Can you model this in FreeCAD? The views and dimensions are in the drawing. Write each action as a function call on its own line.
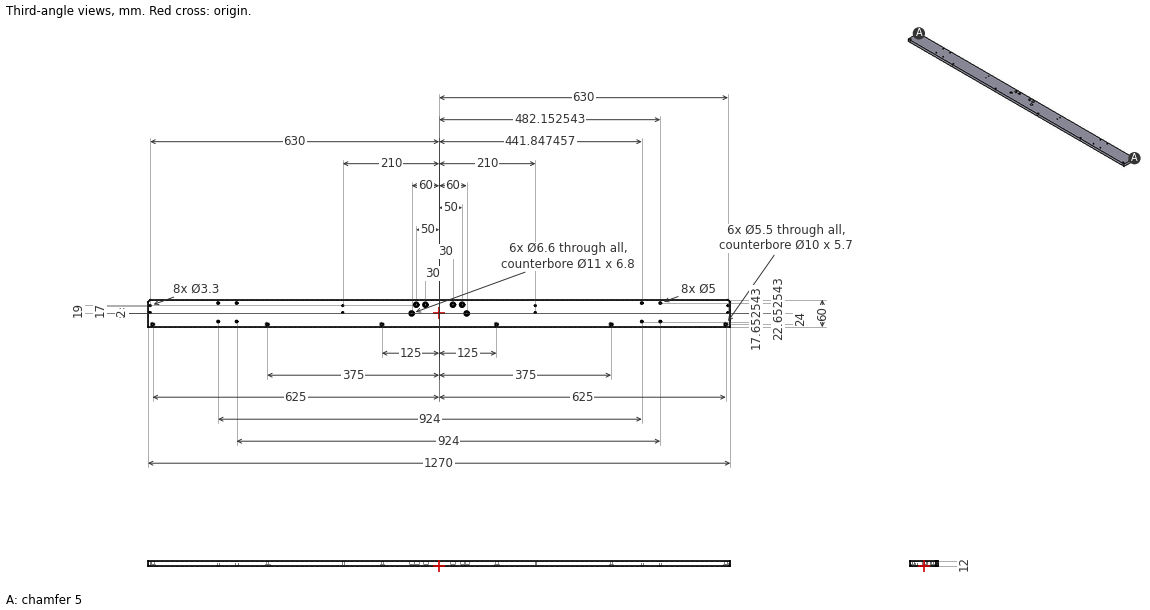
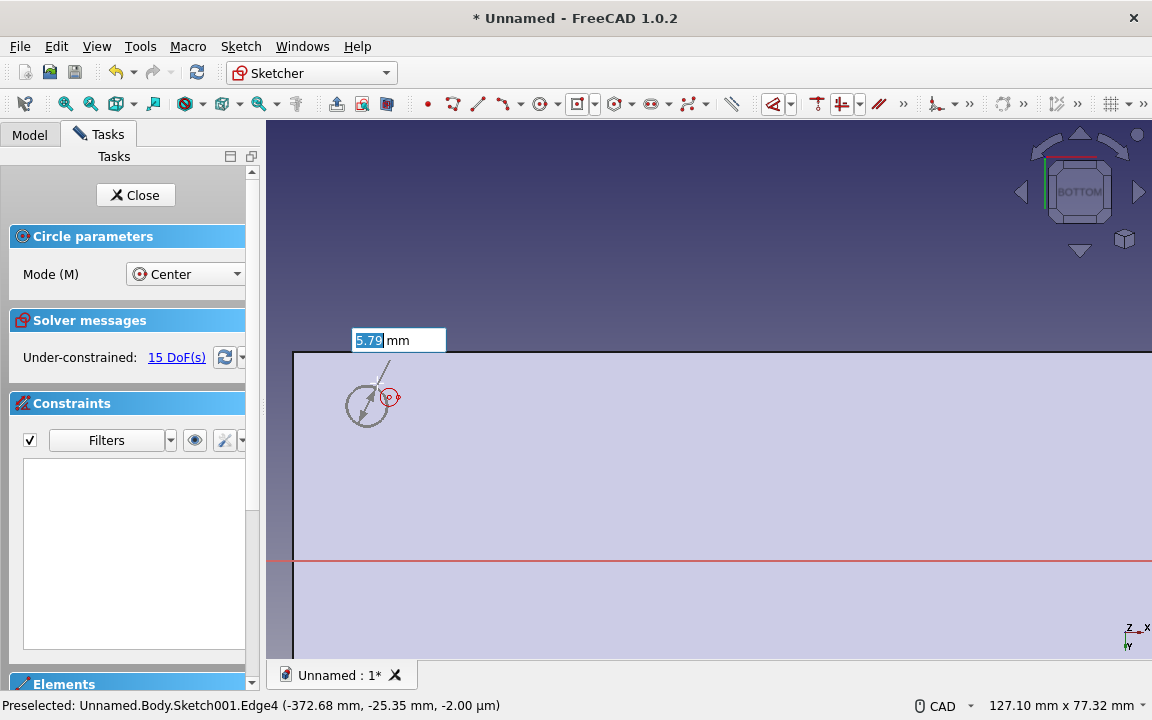
click(376, 380)
key(Escape)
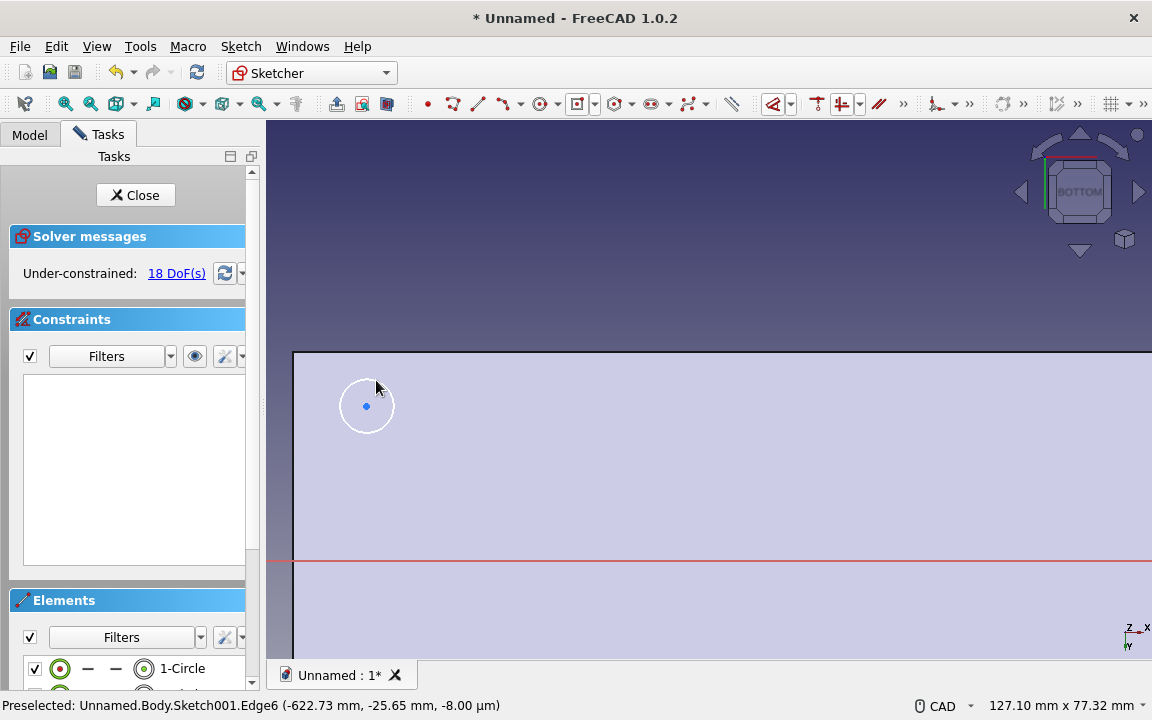
scroll(376, 384, down, 14)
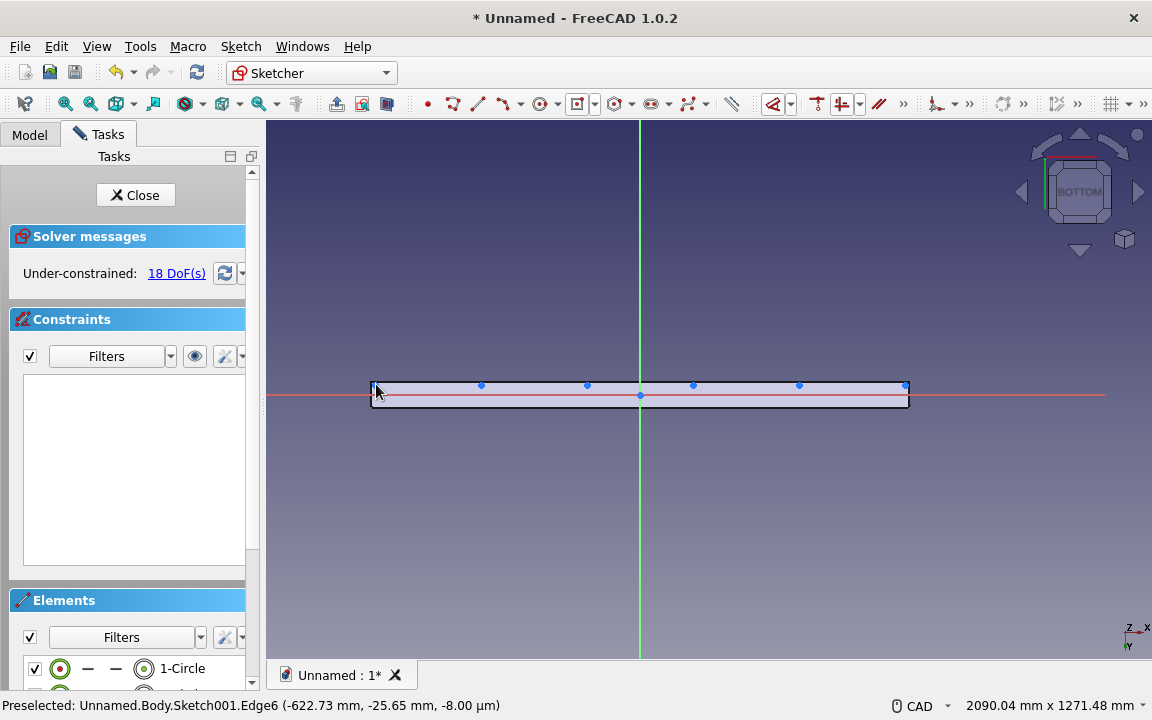
scroll(906, 384, up, 12)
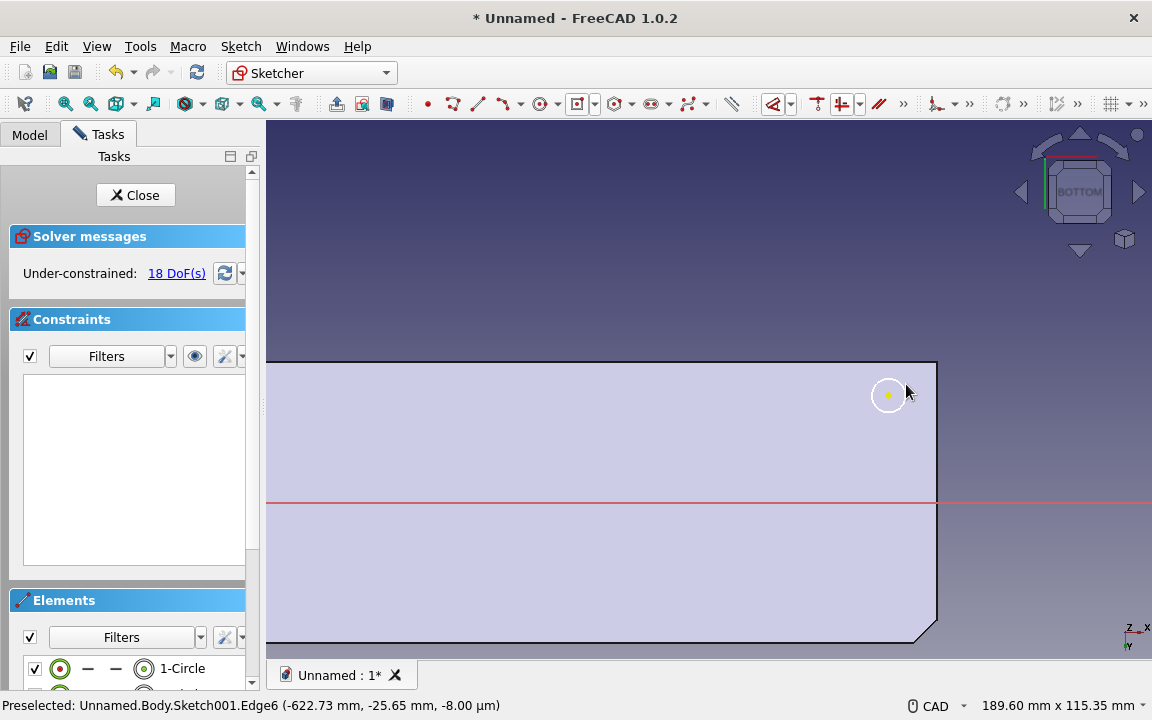
click(901, 384)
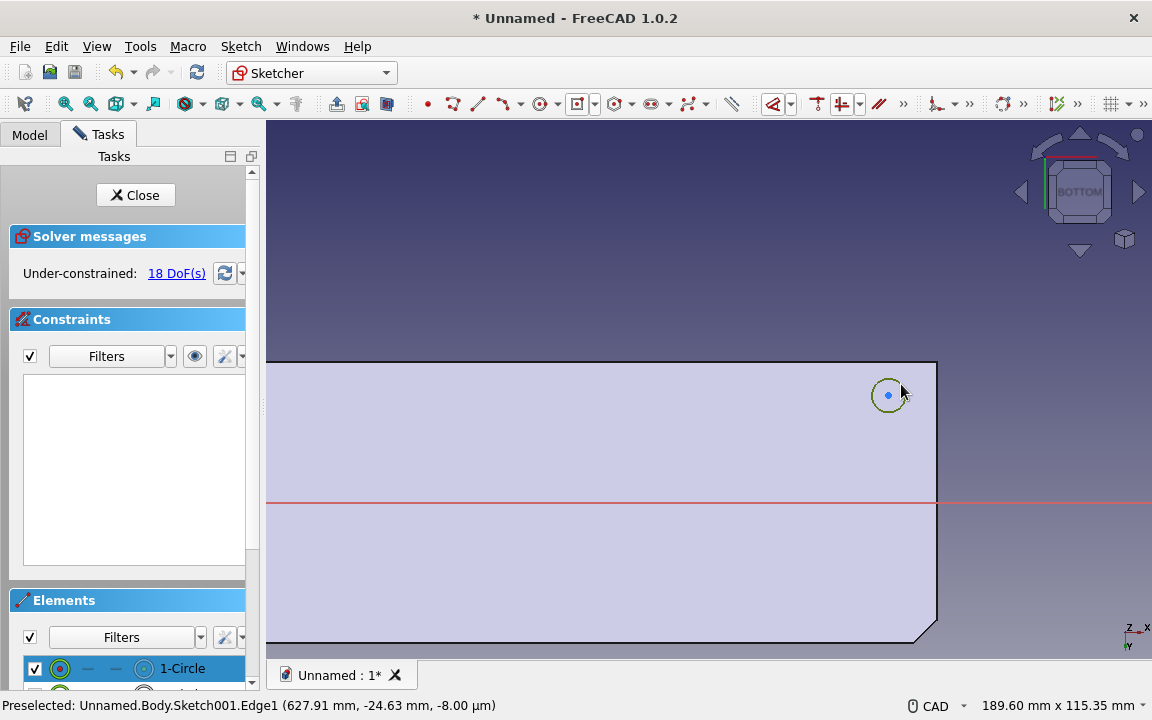
scroll(907, 384, down, 12)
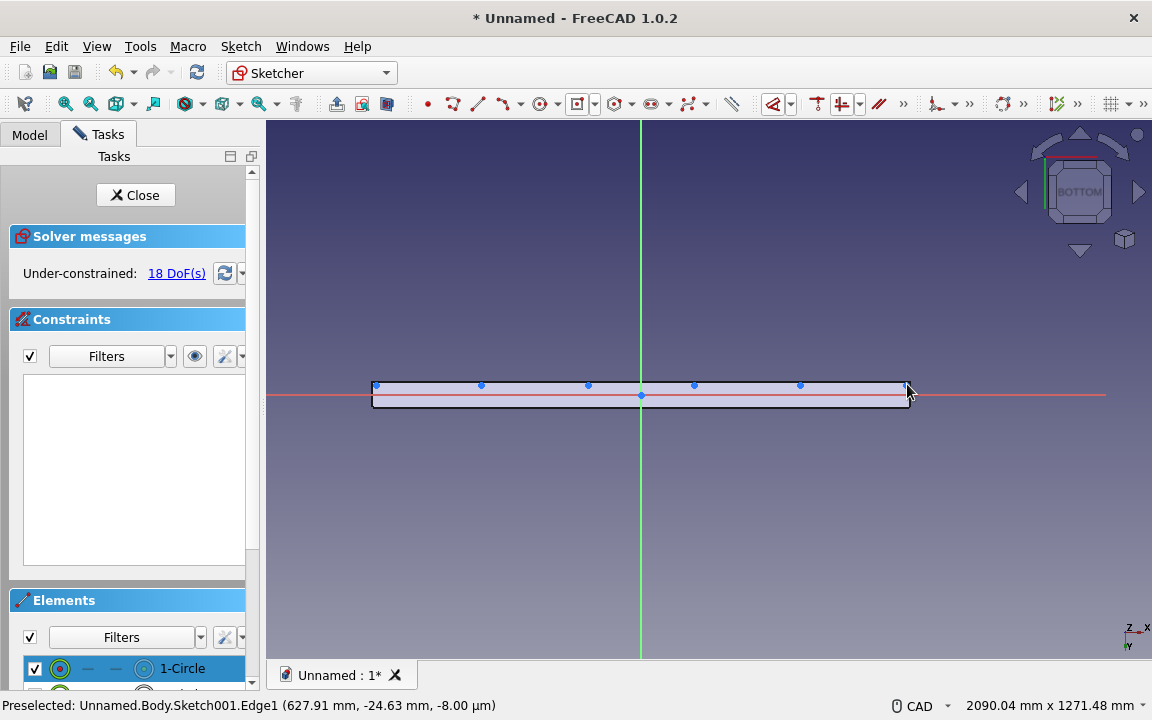
scroll(801, 384, up, 12)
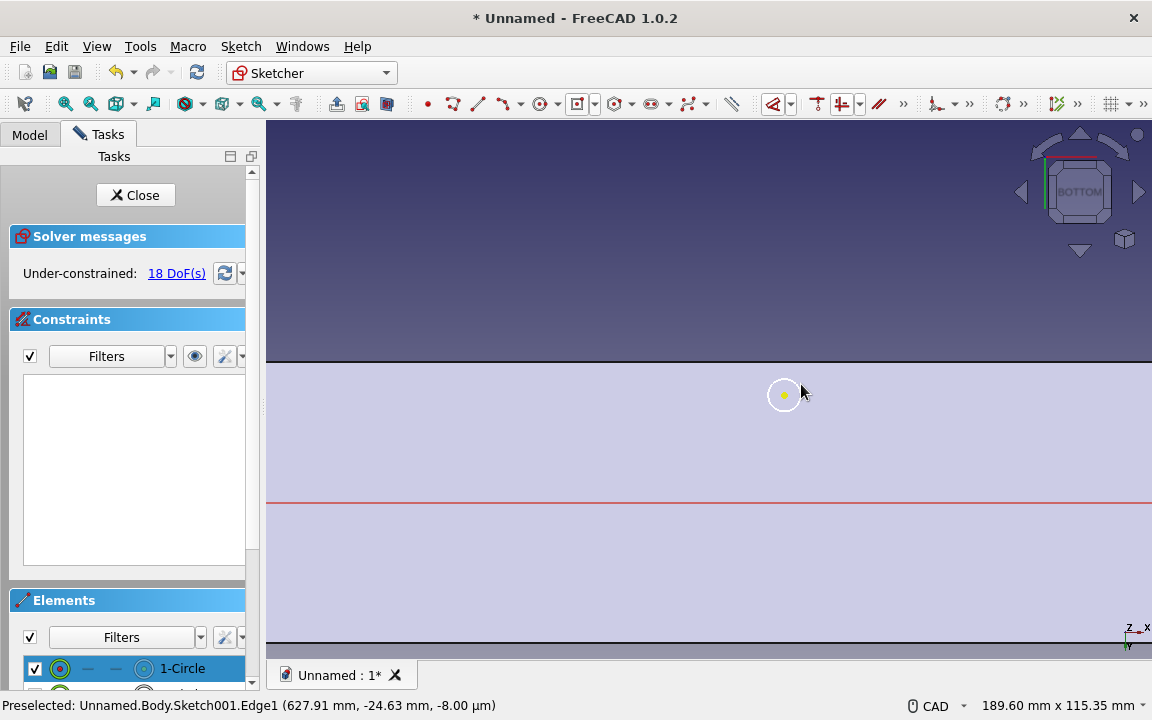
click(796, 384)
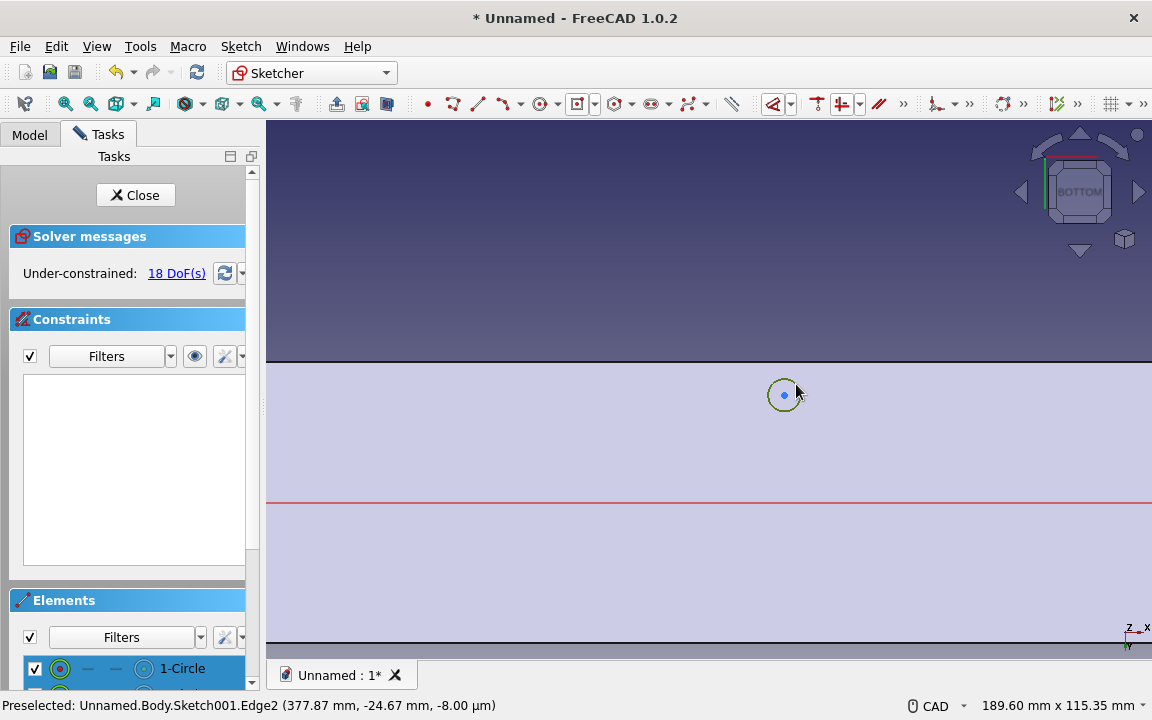
scroll(801, 384, down, 12)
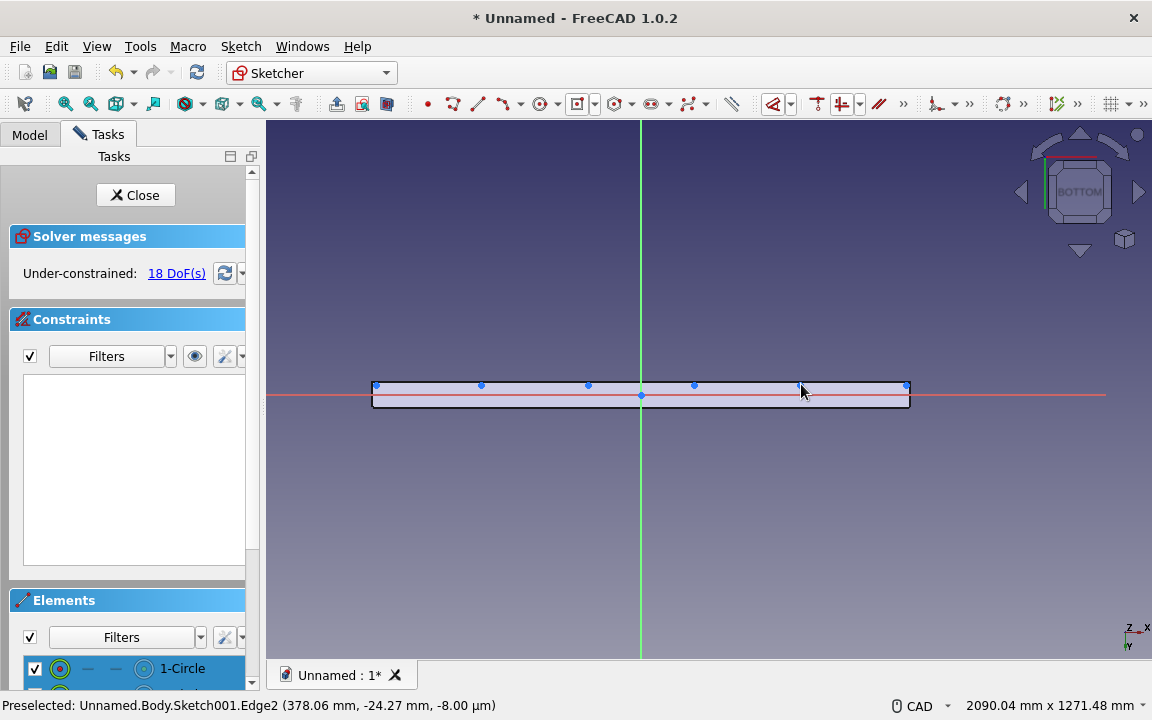
scroll(695, 384, up, 12)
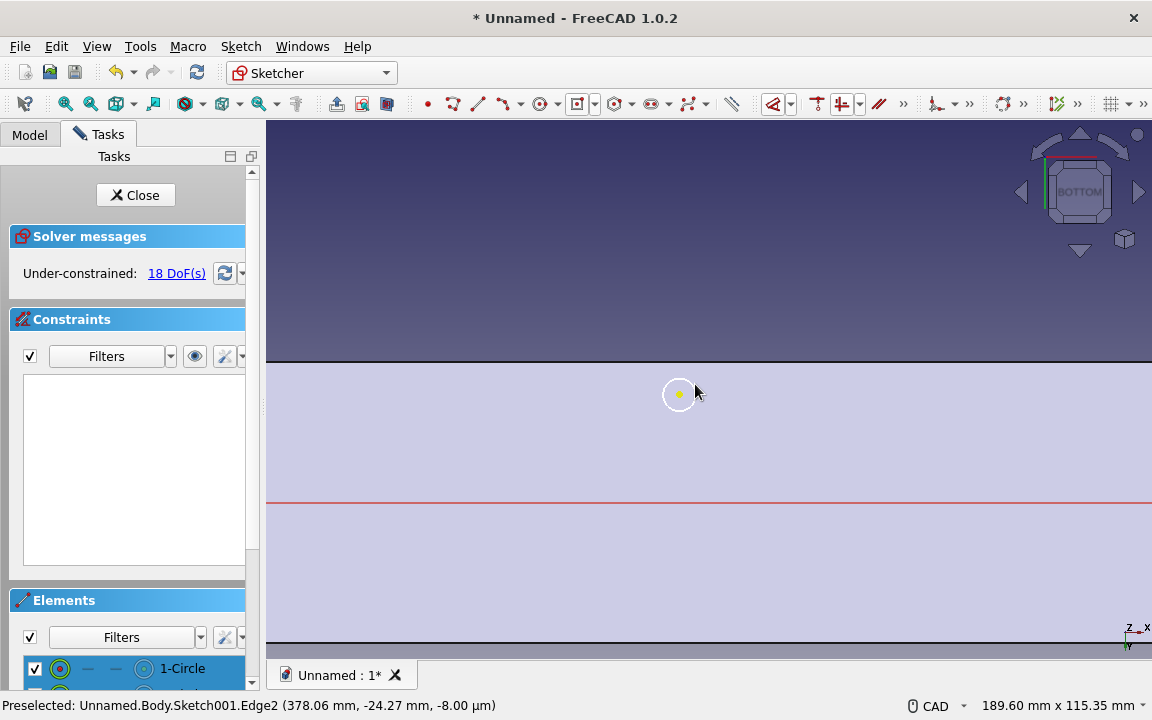
click(691, 383)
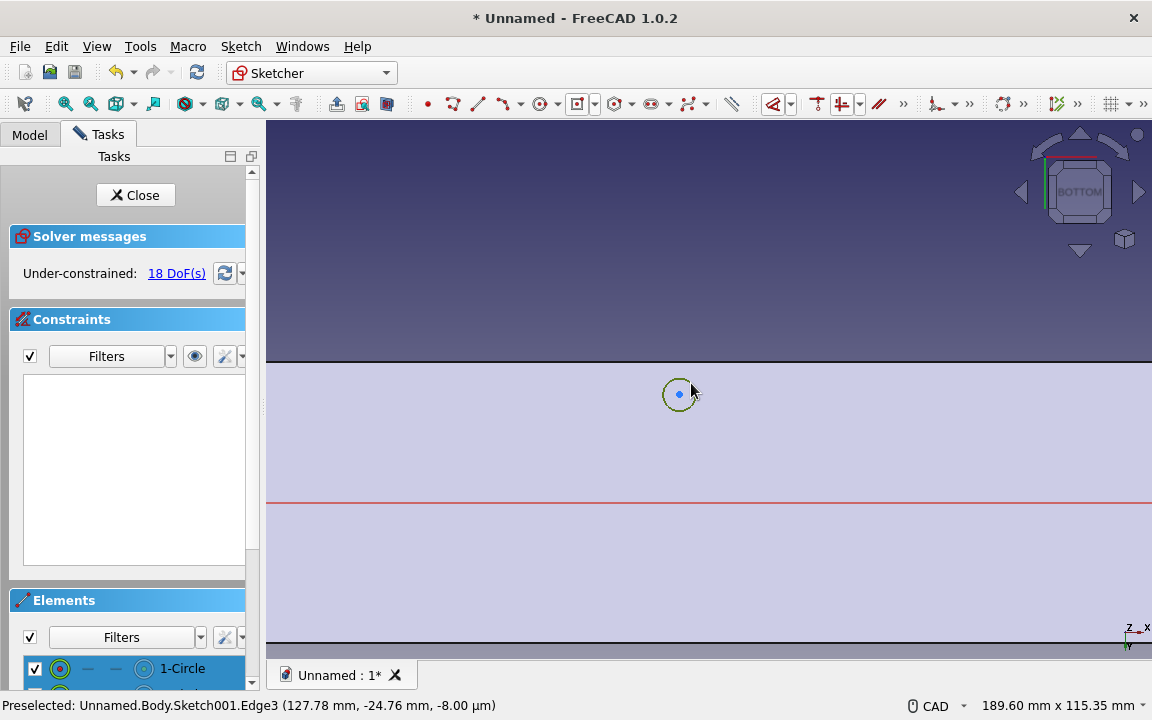
scroll(695, 384, down, 12)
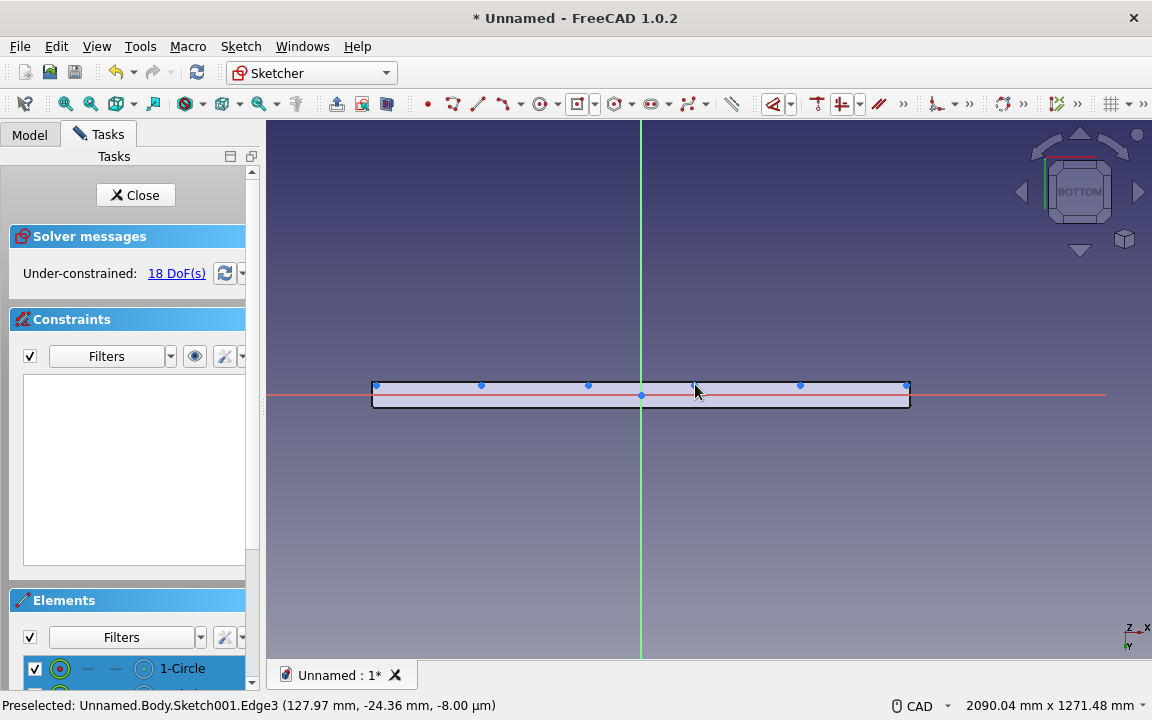
scroll(589, 384, up, 12)